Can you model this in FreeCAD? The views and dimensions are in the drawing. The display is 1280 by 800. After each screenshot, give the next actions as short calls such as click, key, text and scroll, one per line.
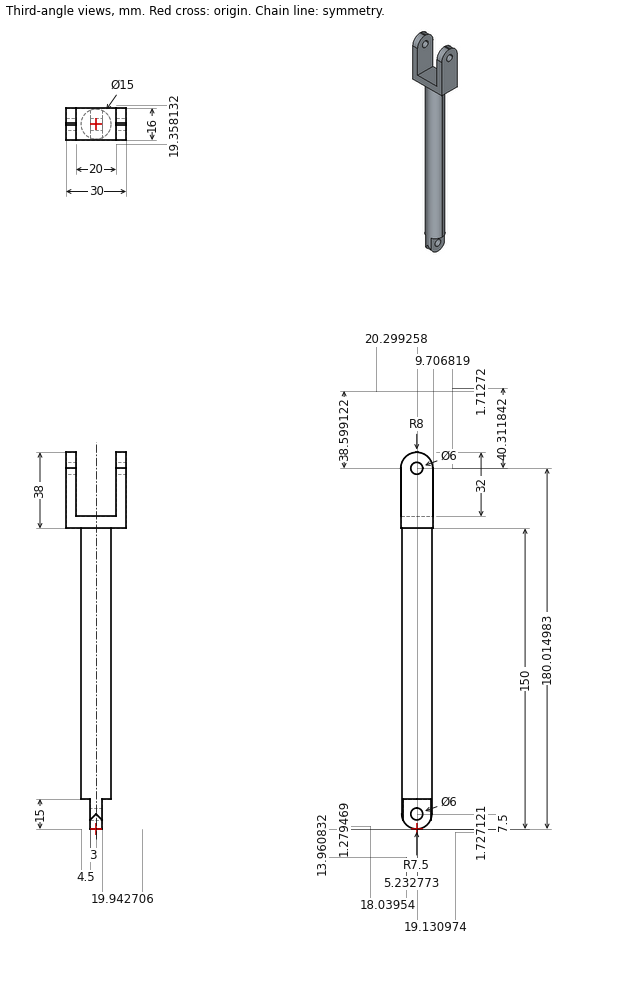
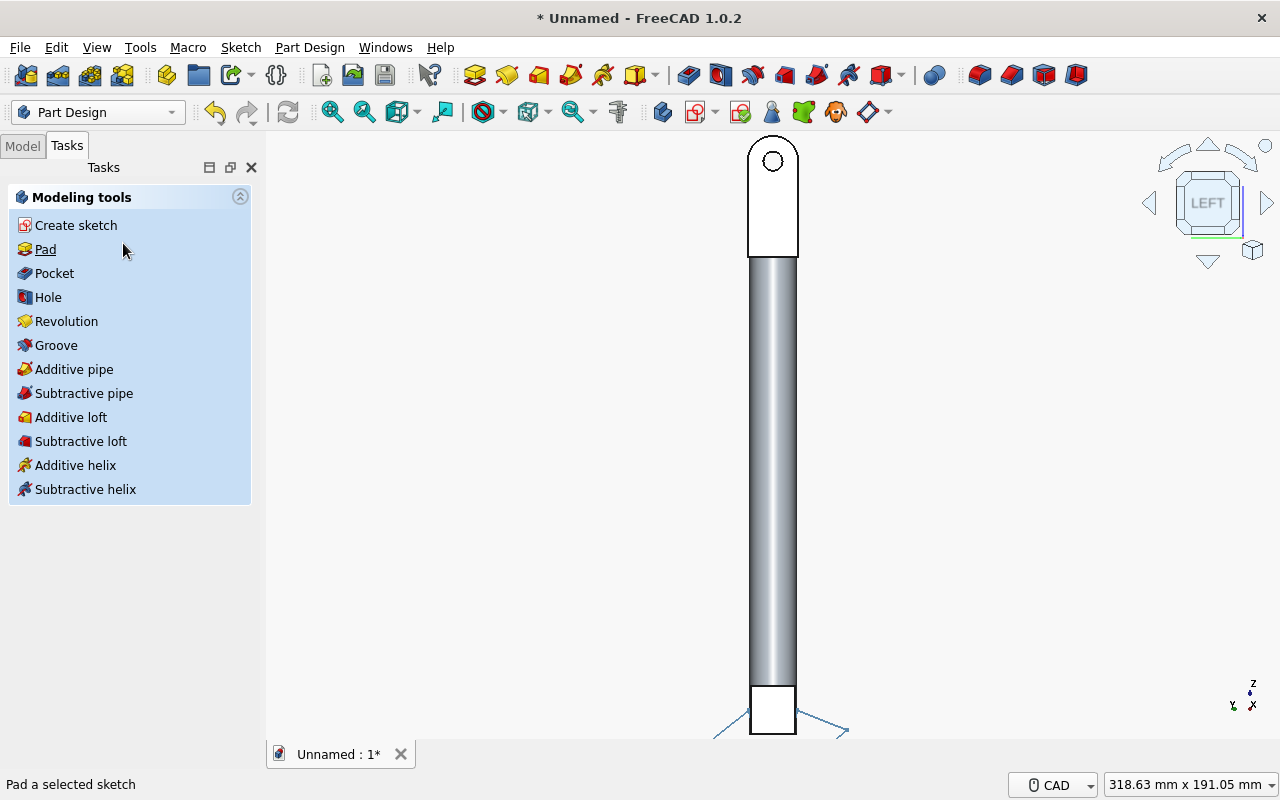
click(690, 76)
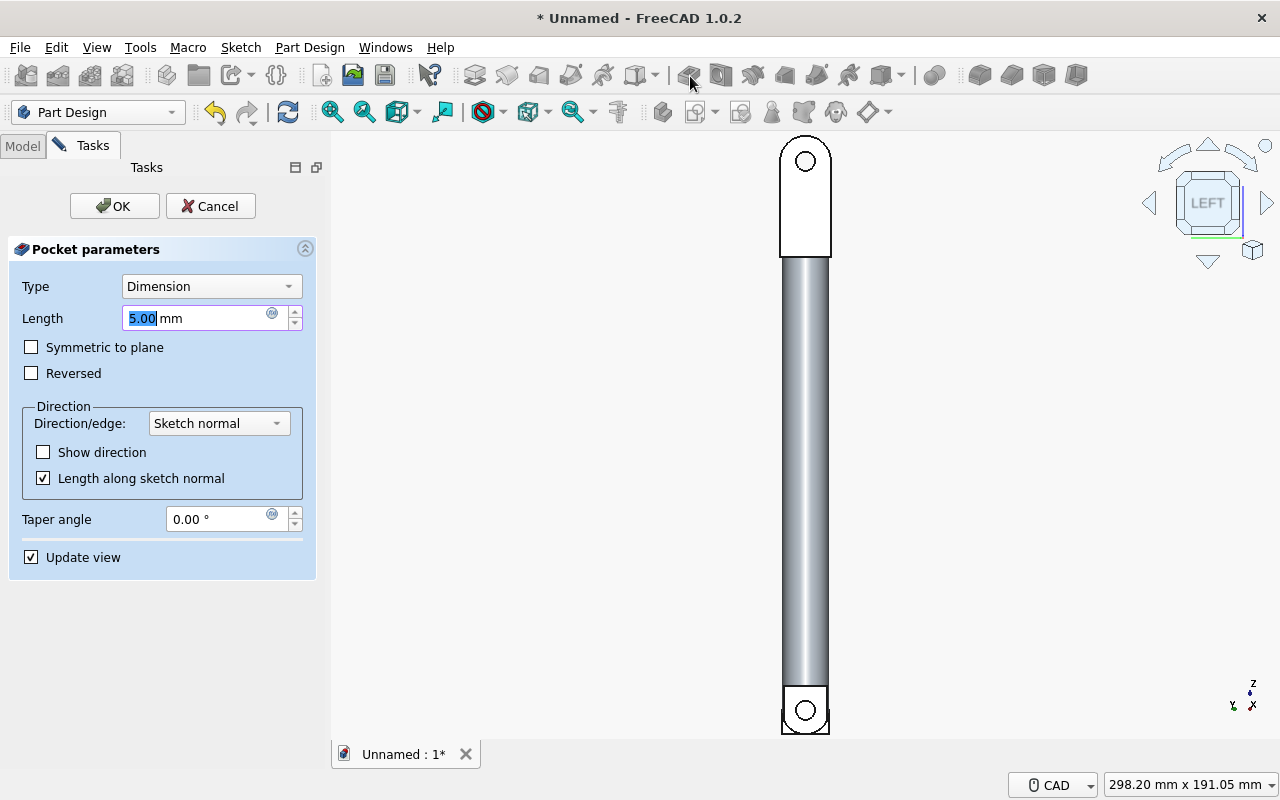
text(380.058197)
key(Tab)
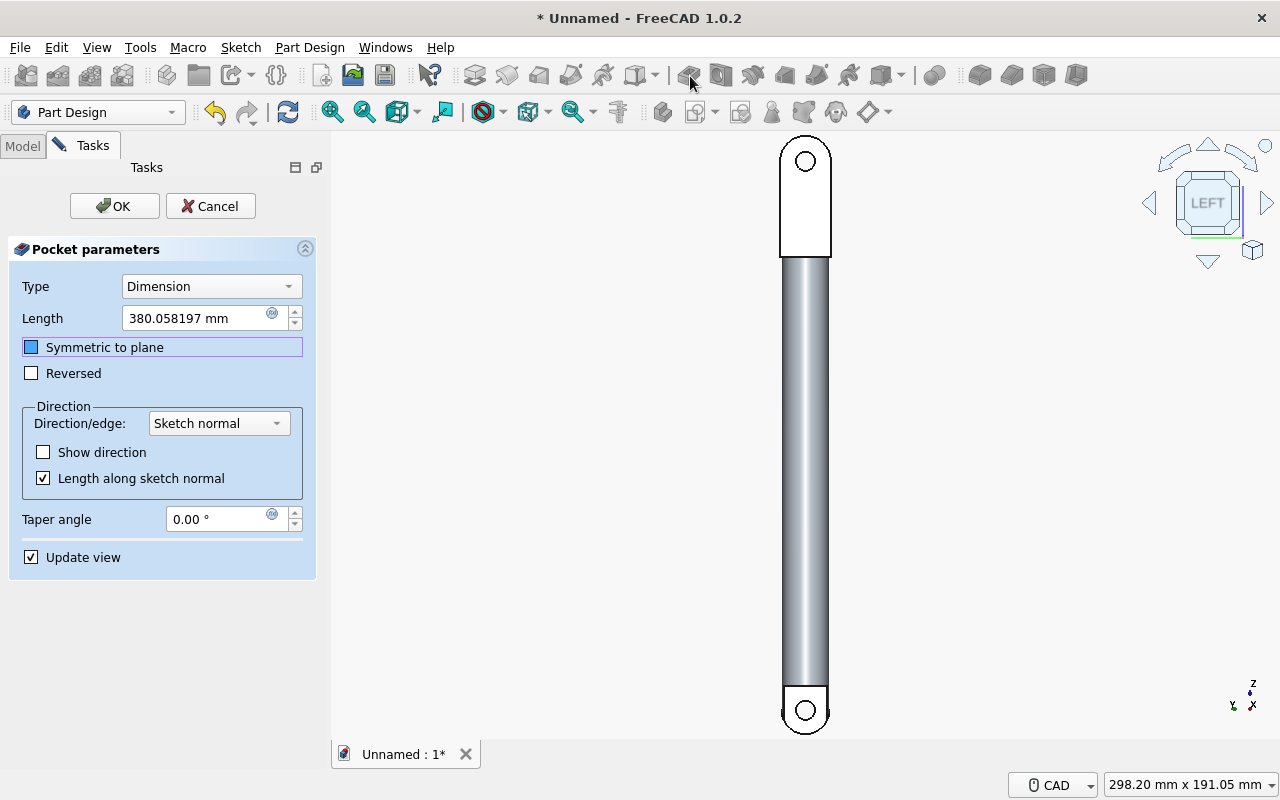
click(30, 347)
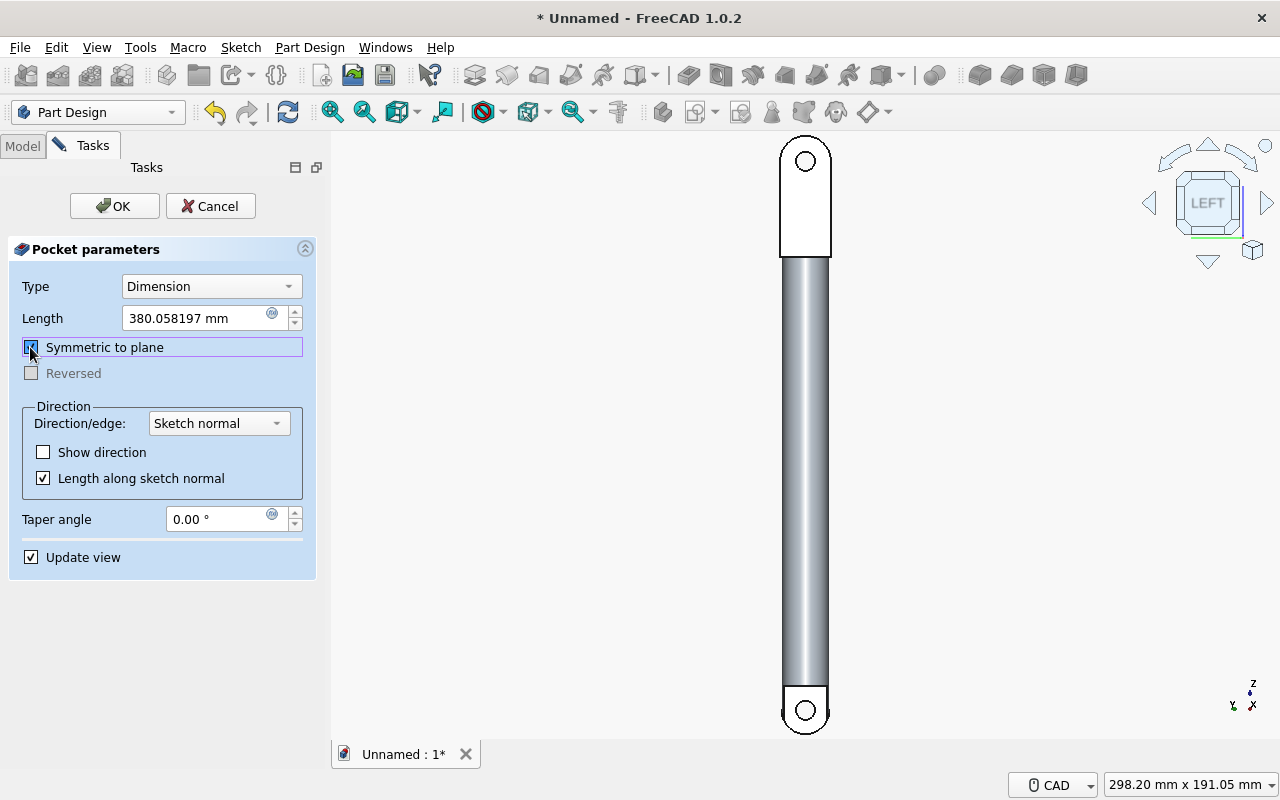
click(115, 206)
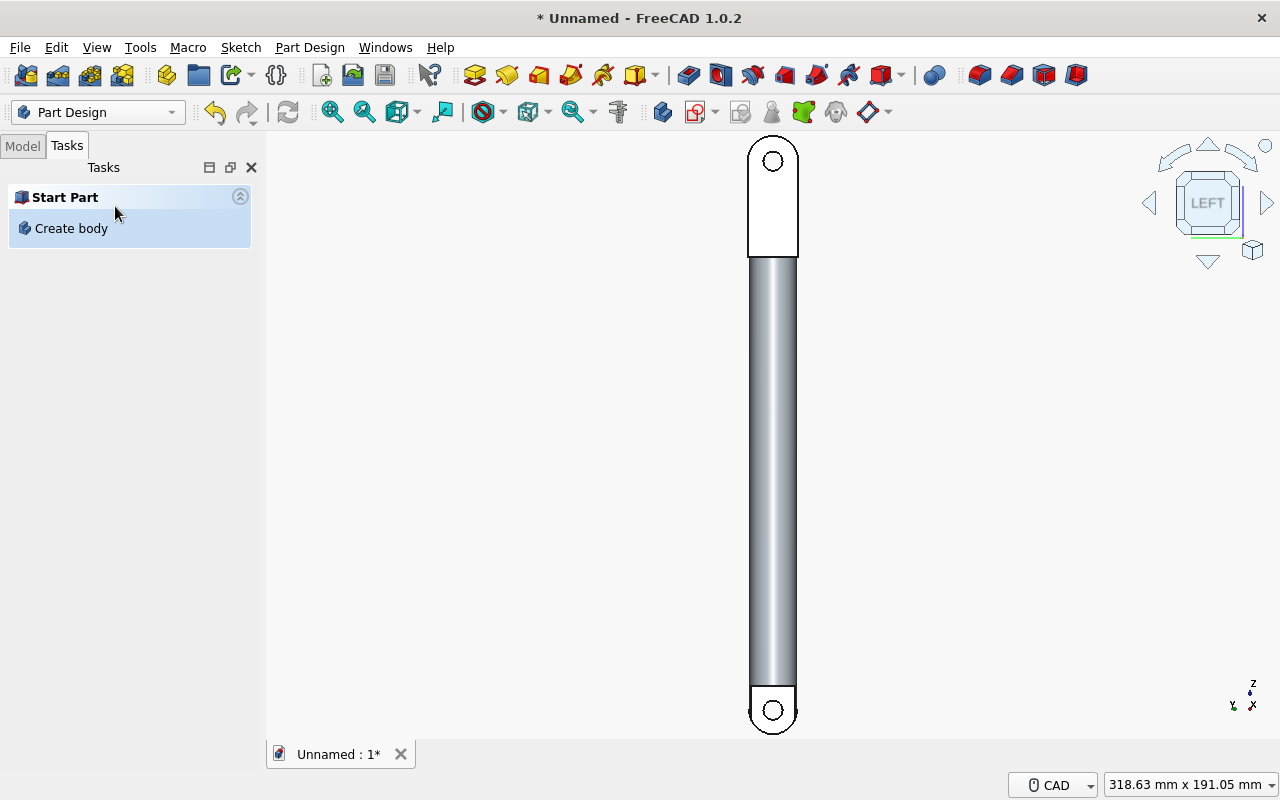
key(0)